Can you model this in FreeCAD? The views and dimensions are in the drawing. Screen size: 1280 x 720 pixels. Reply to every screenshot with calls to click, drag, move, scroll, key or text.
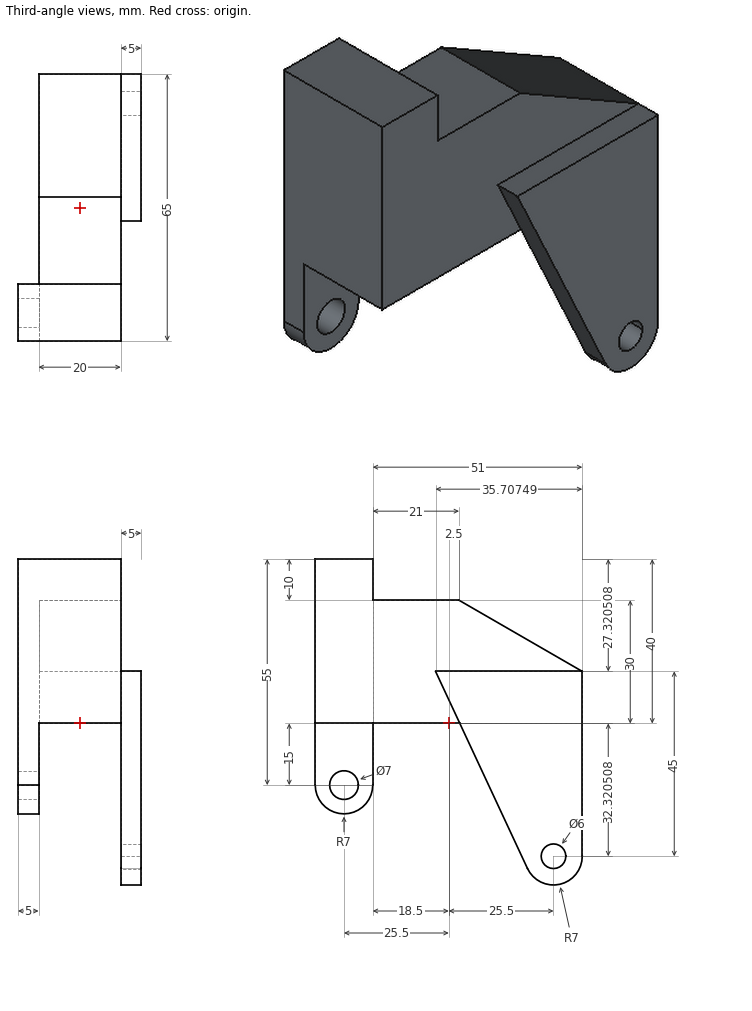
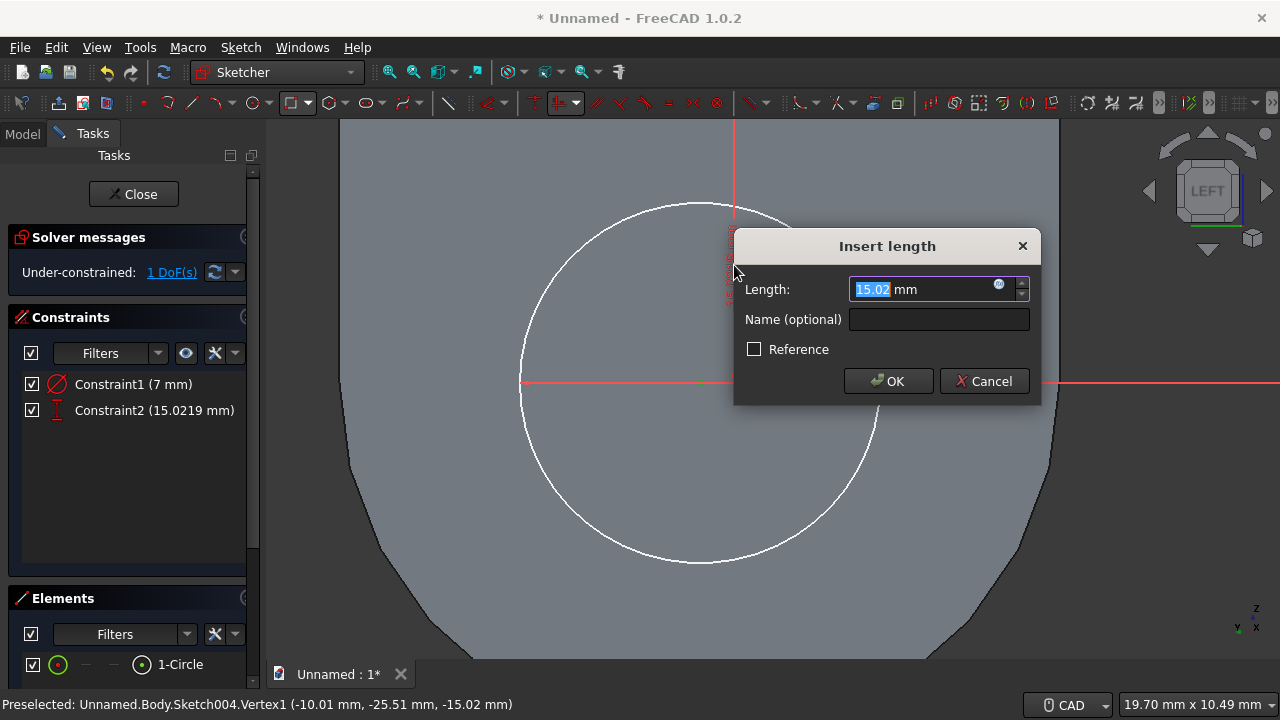
text(15)
key(Return)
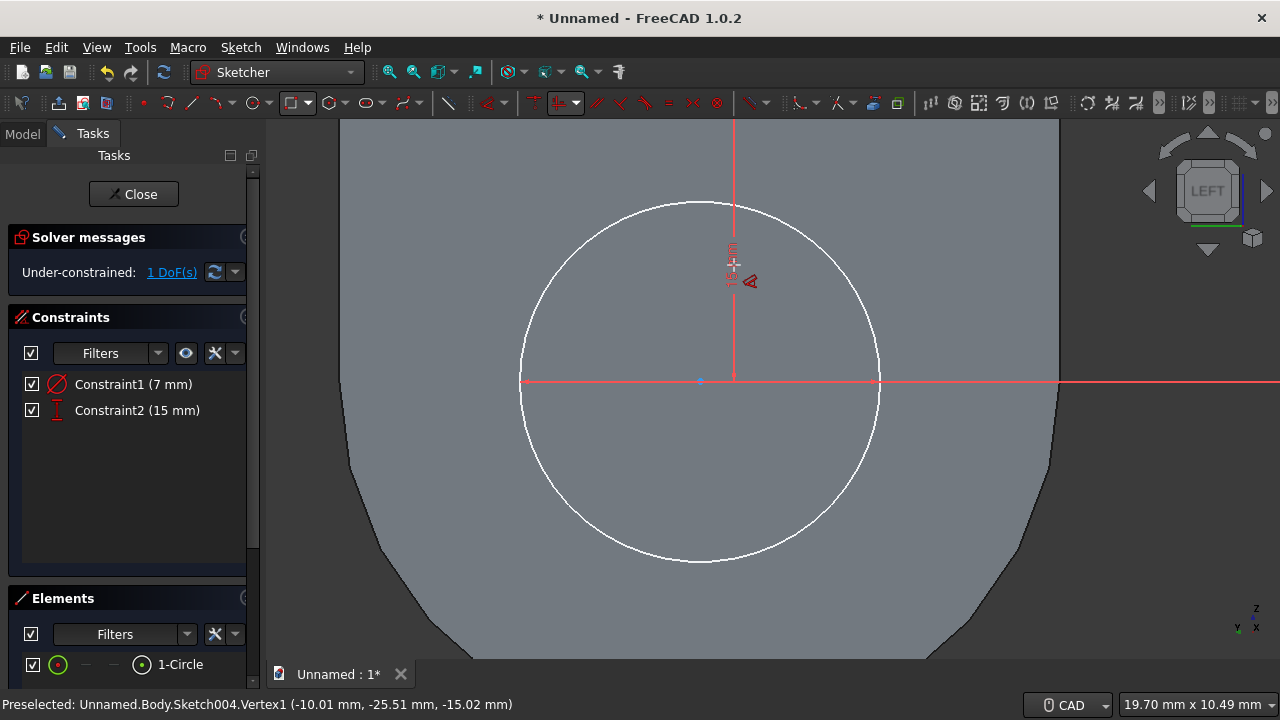
click(700, 382)
click(497, 416)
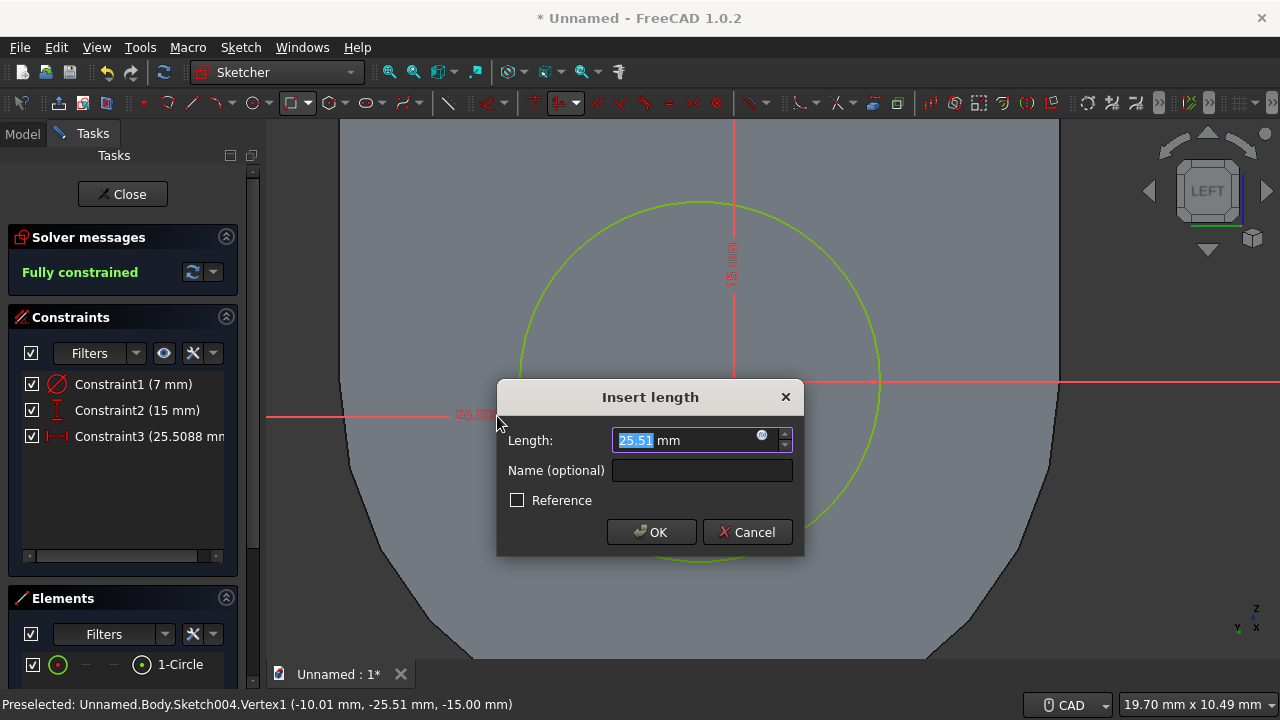
text(25.5)
key(Return)
key(Escape)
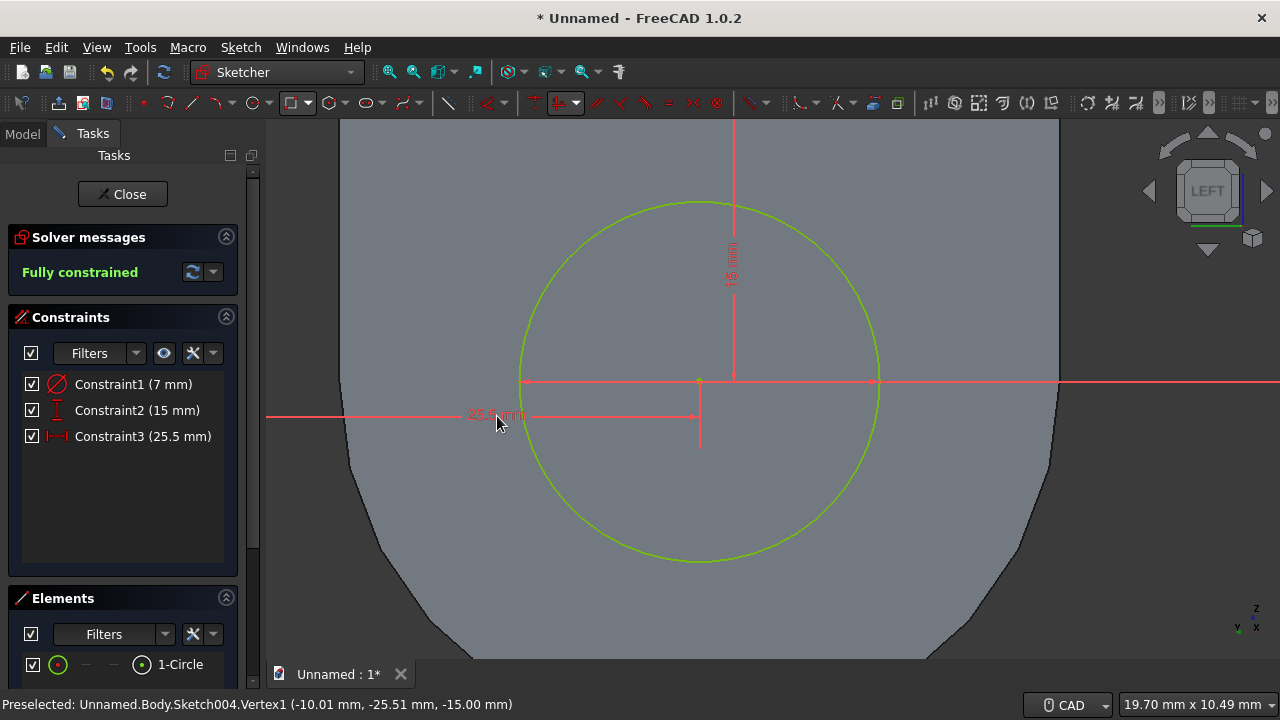
click(123, 194)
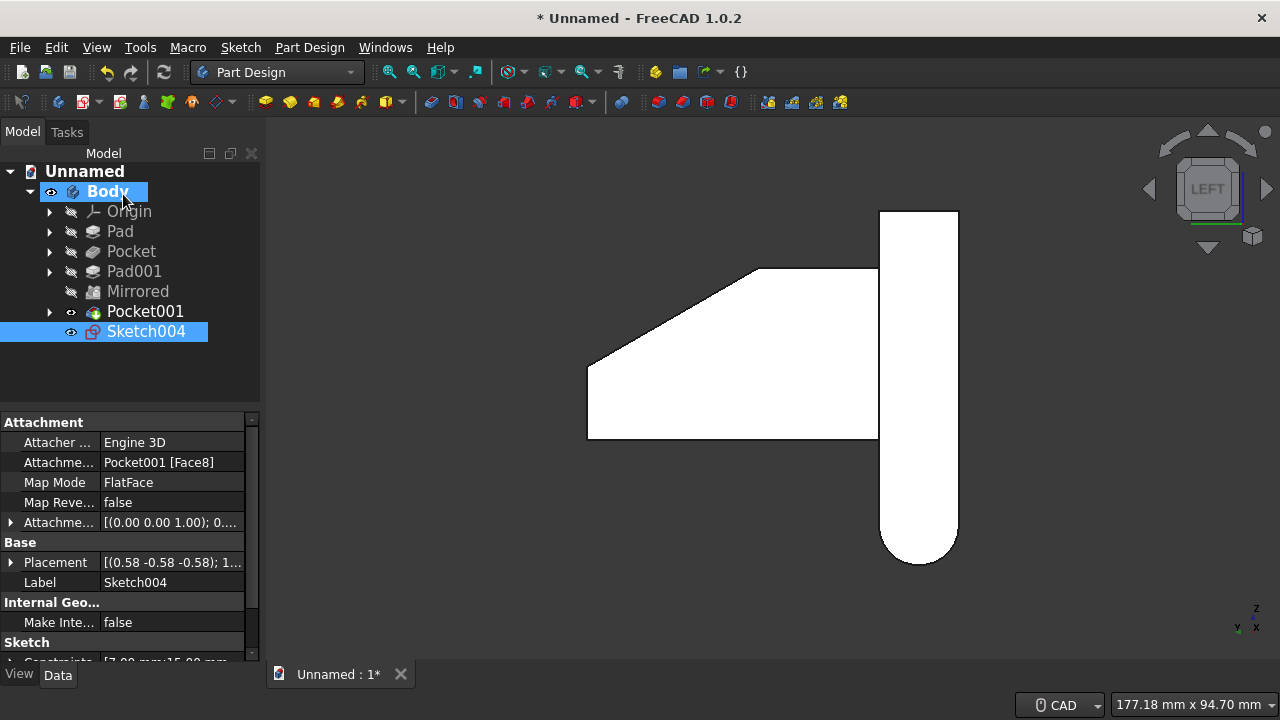
click(432, 102)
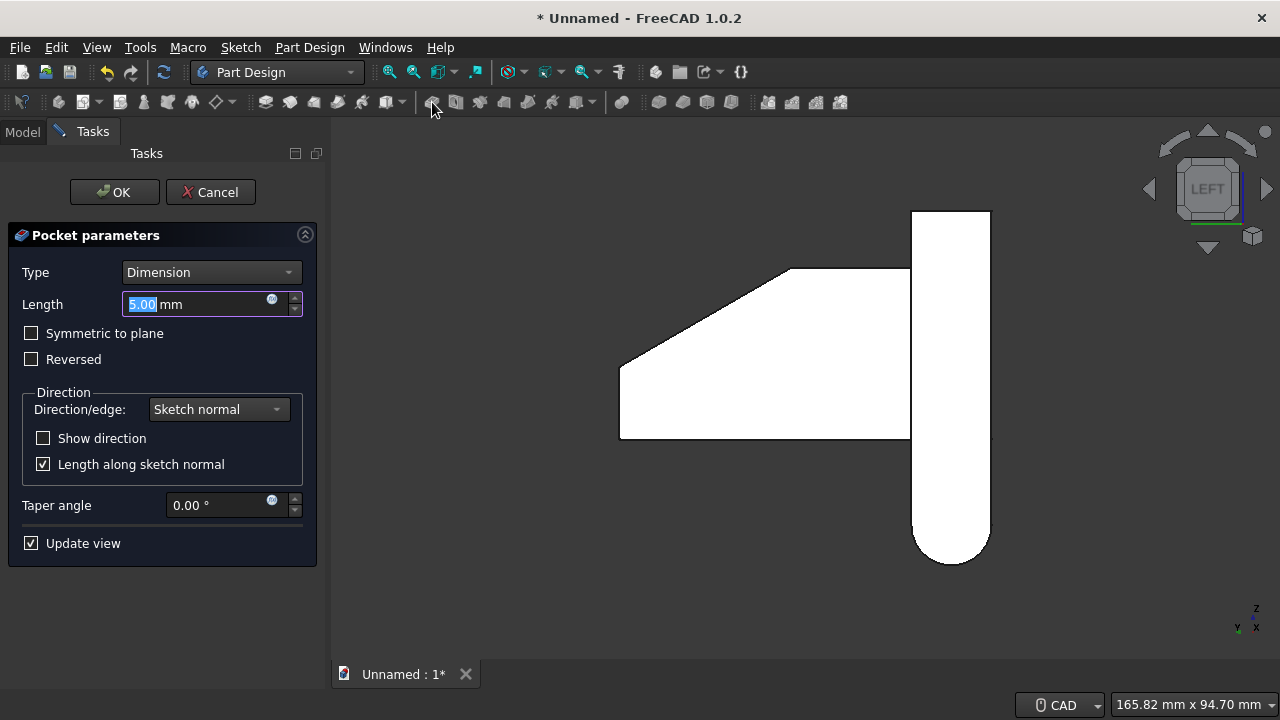
text(5)
key(Tab)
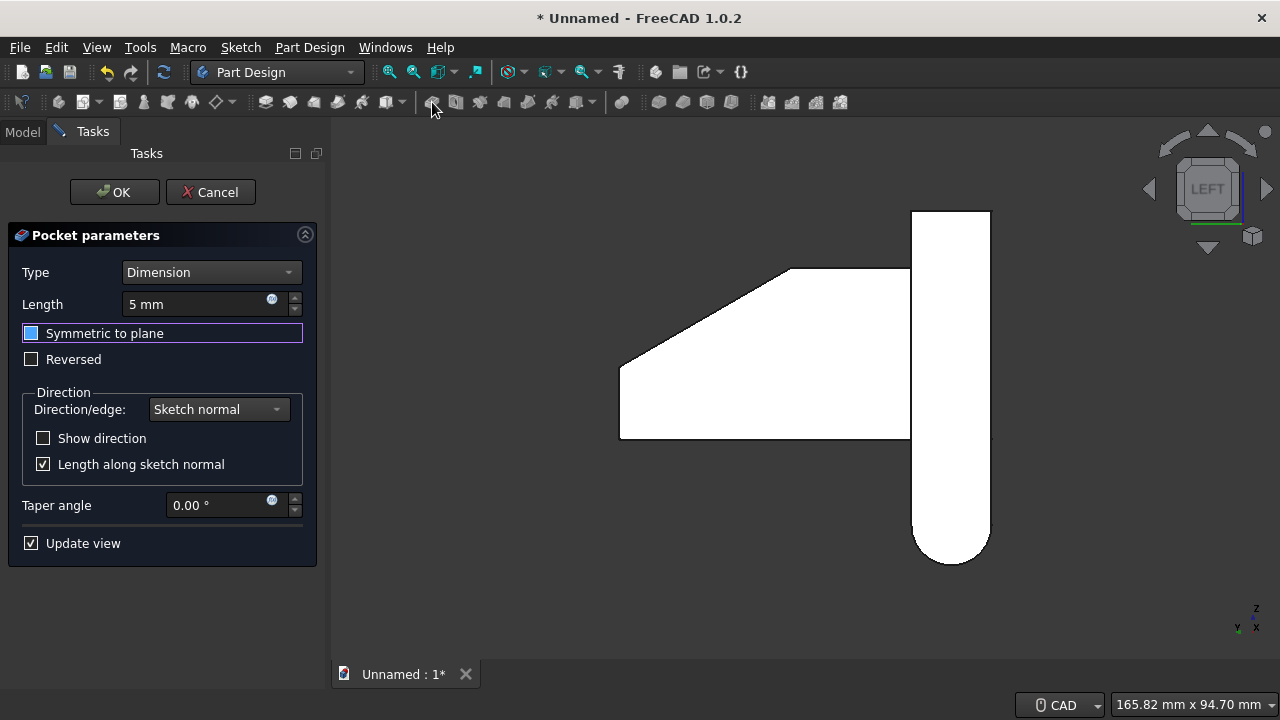
click(30, 359)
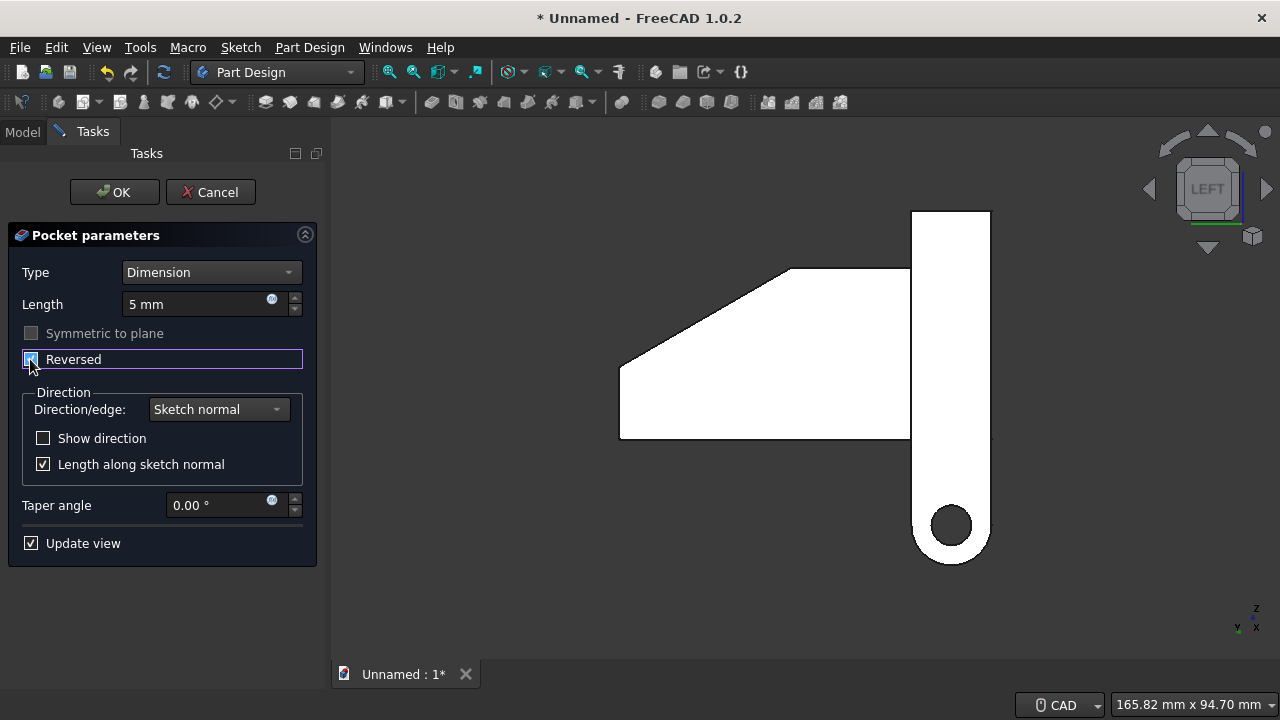
click(115, 192)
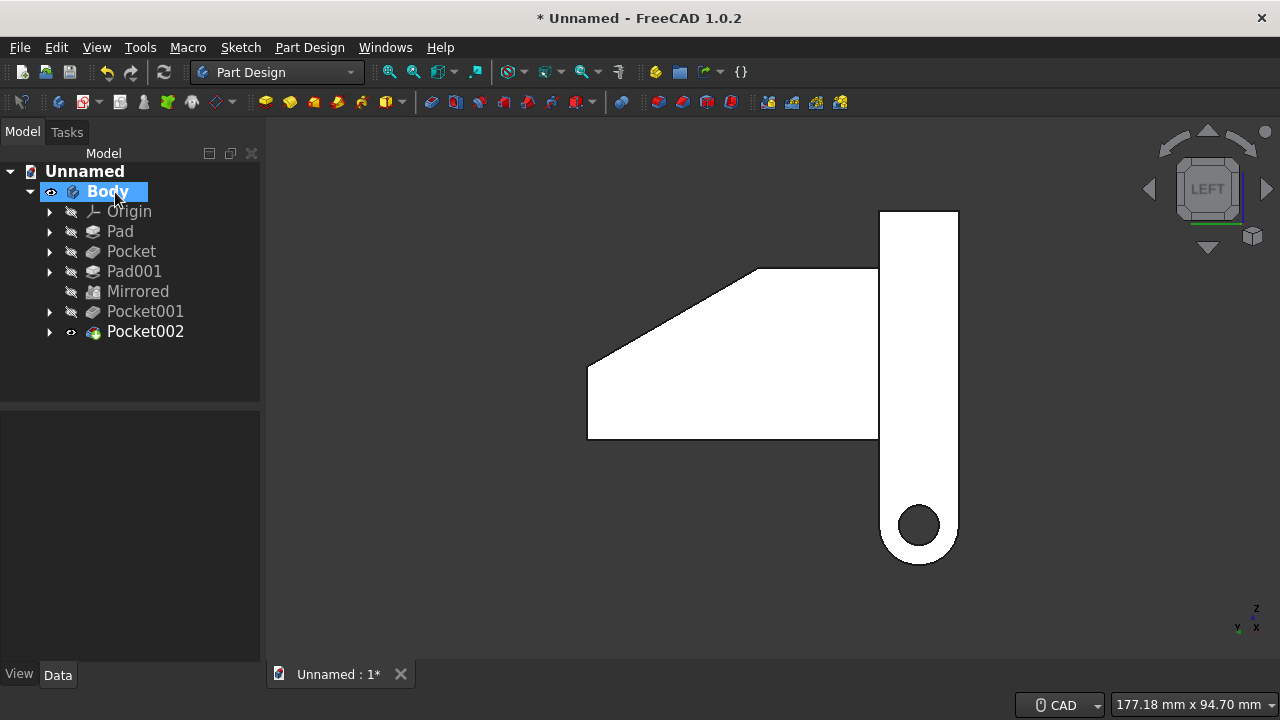
key(0)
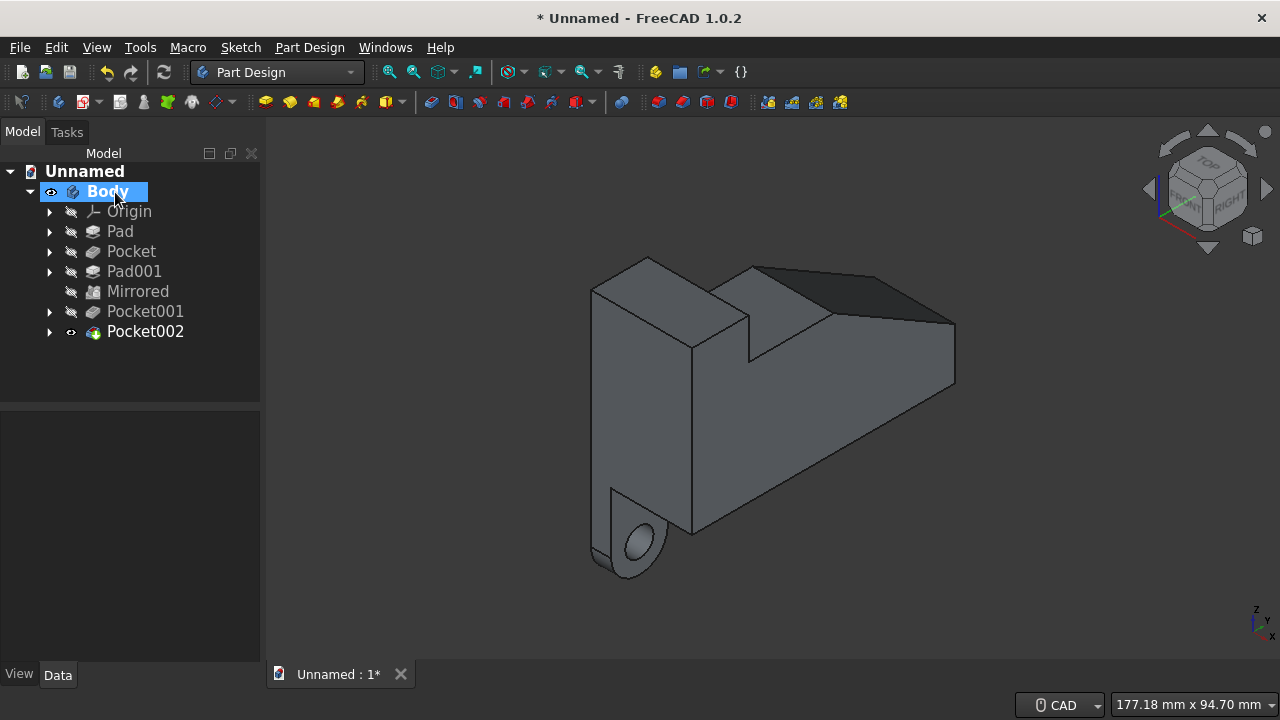
click(824, 392)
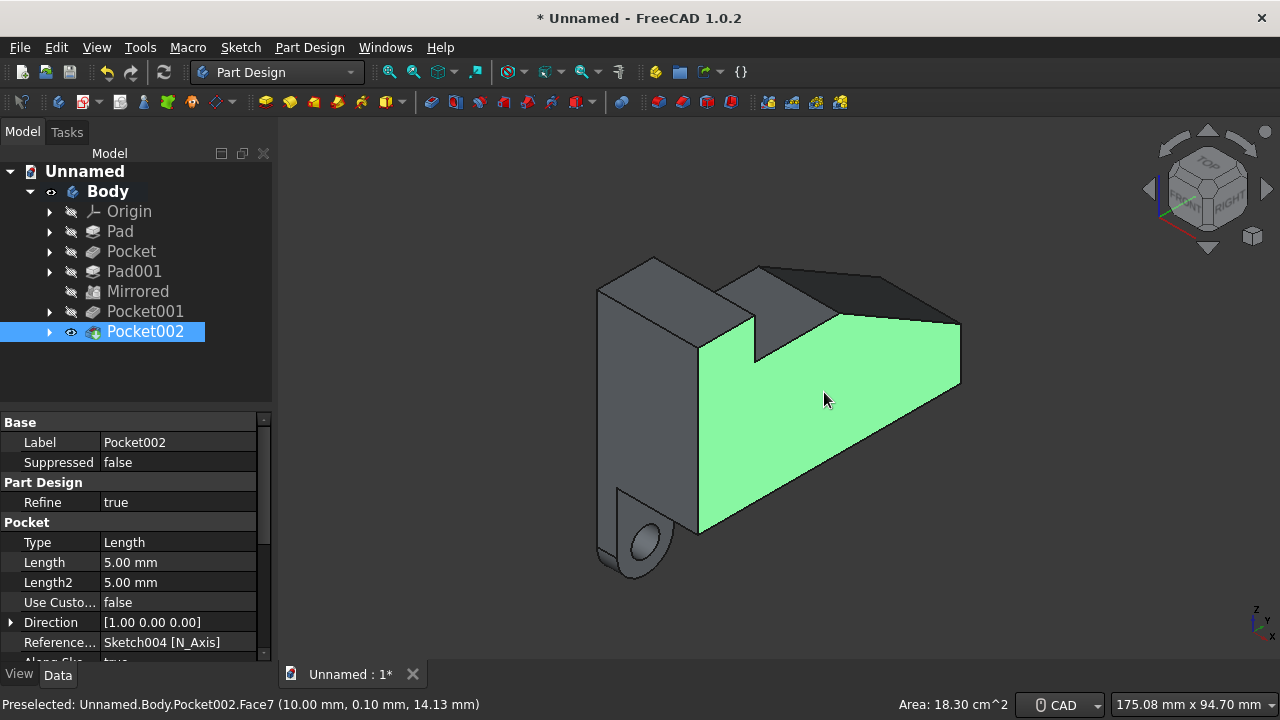
click(84, 102)